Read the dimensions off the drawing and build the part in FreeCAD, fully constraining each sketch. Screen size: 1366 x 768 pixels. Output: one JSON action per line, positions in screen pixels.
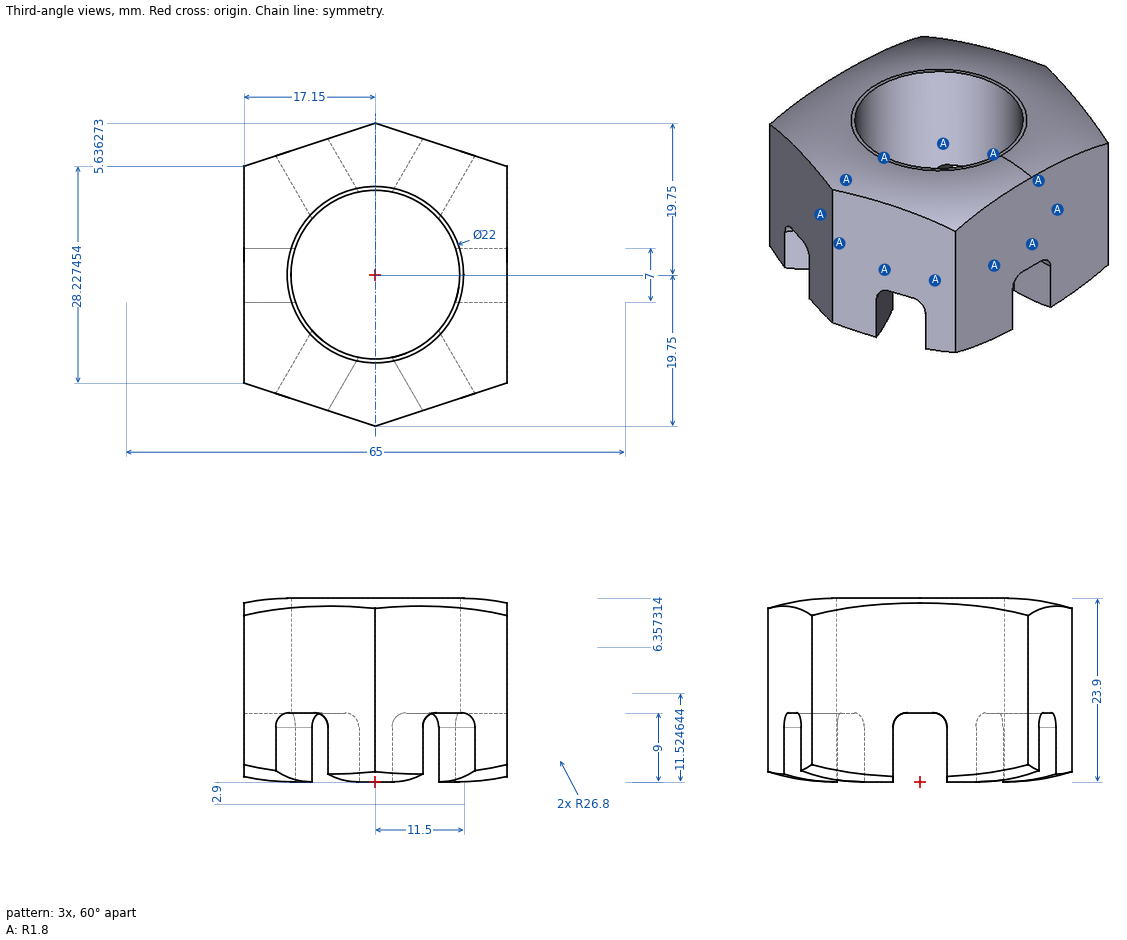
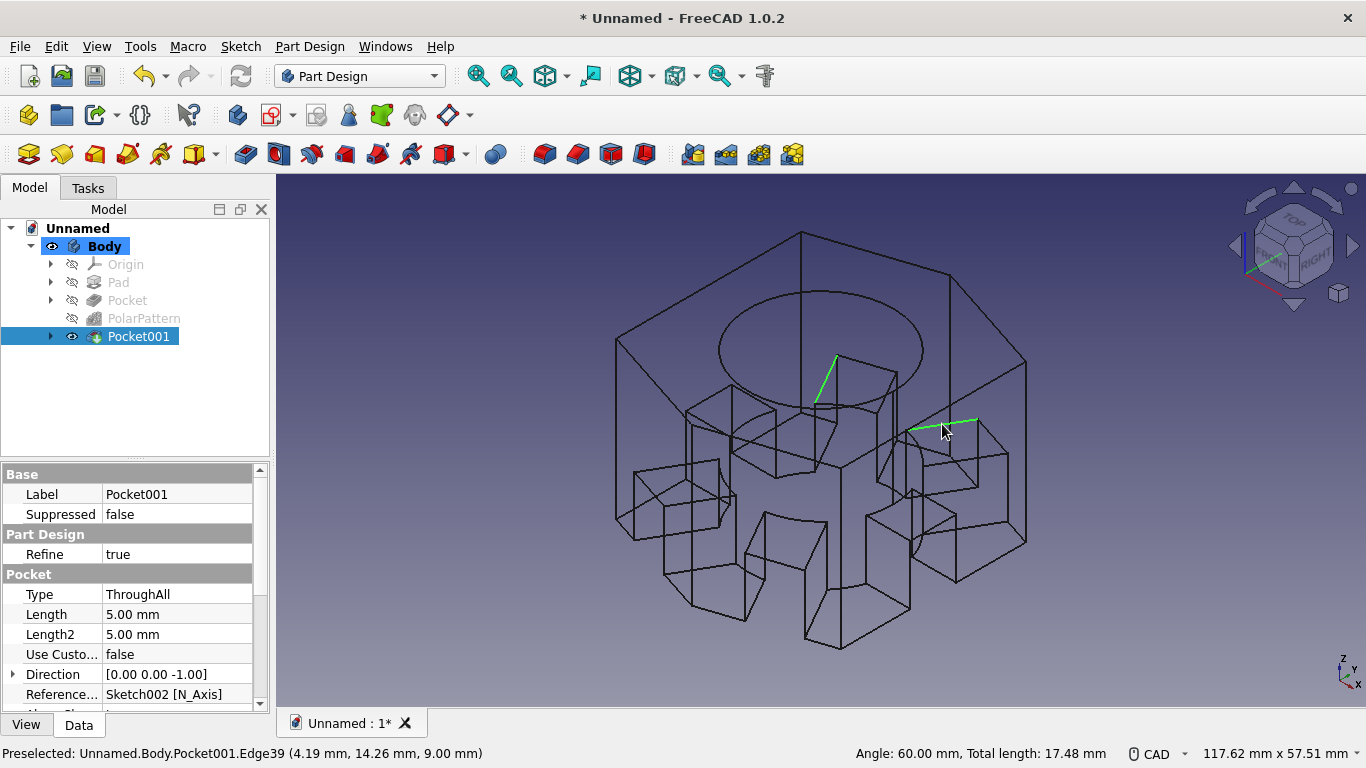
{"action": "left_click", "coordinate": [700, 500], "text": "ctrl"}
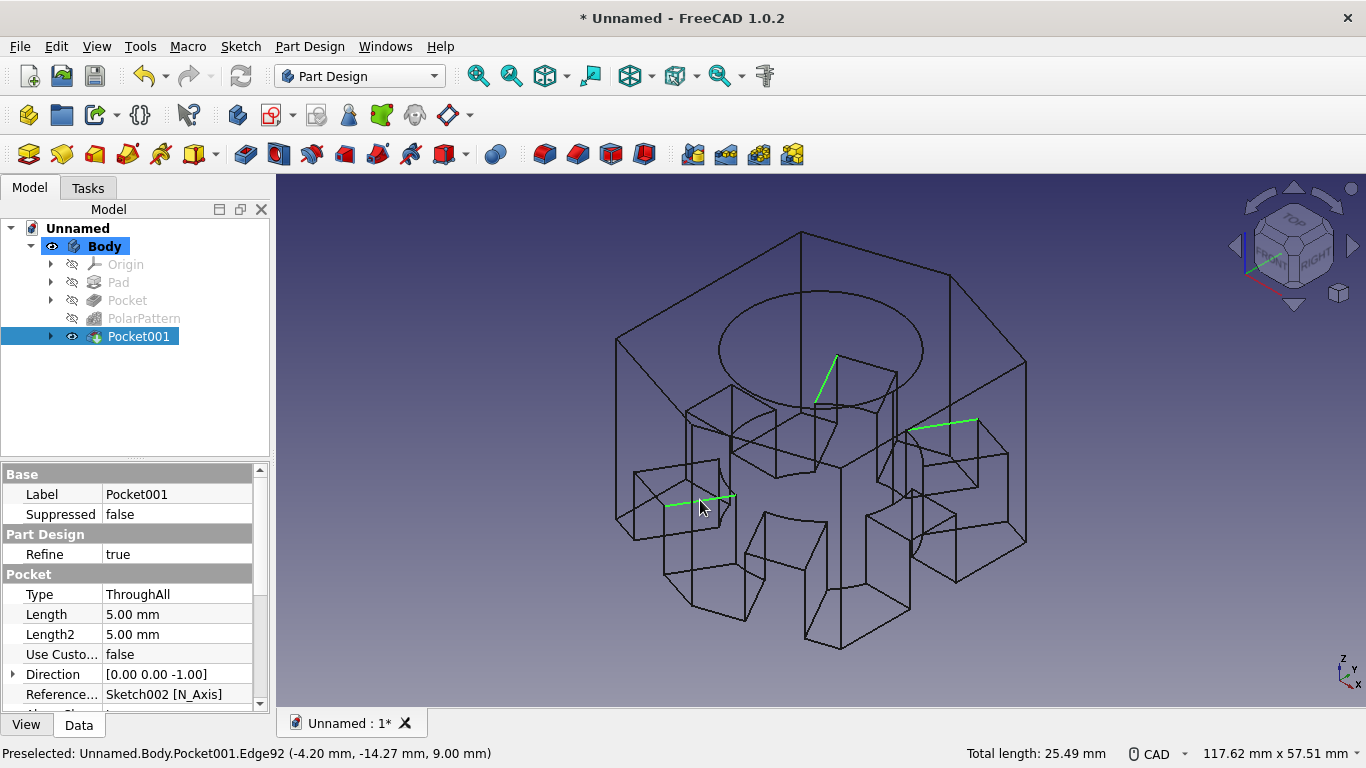
{"action": "left_click", "coordinate": [816, 545], "text": "ctrl"}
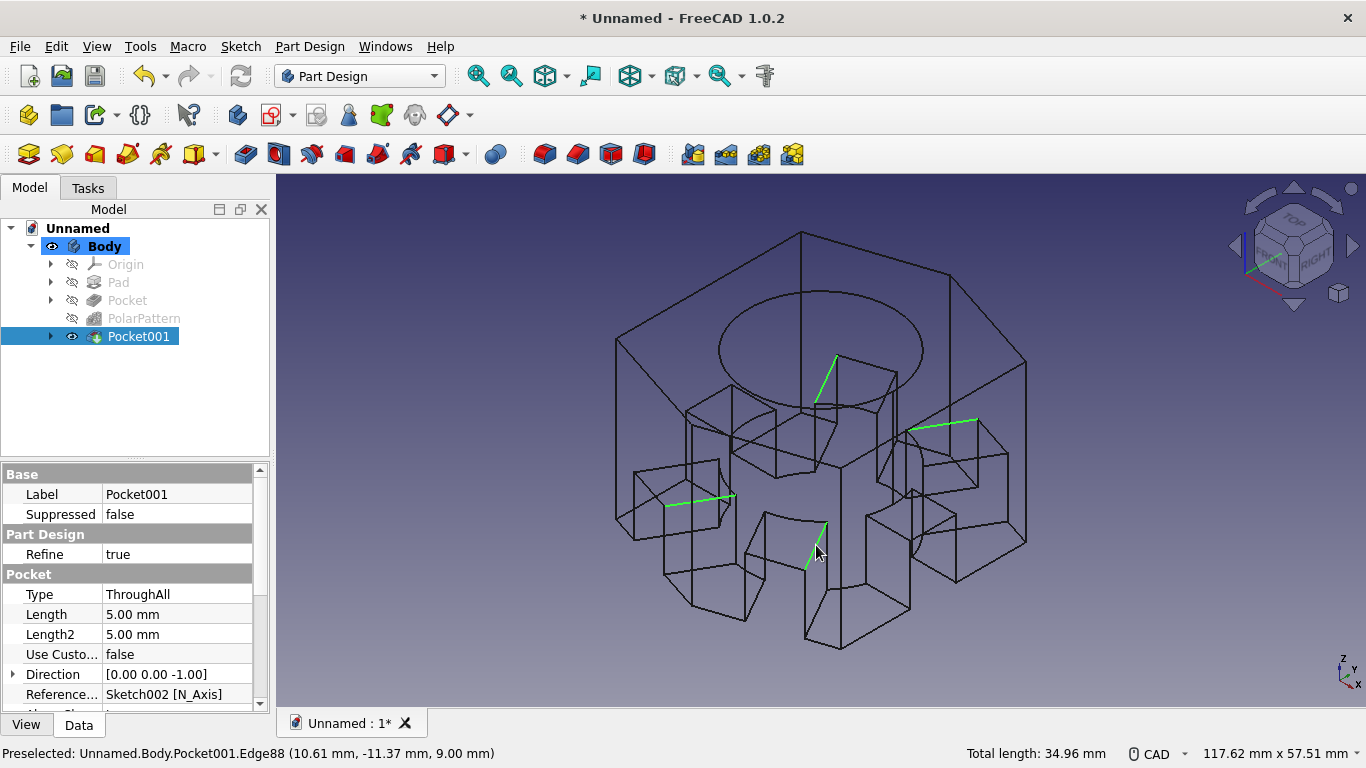
{"action": "left_click", "coordinate": [703, 420], "text": "ctrl"}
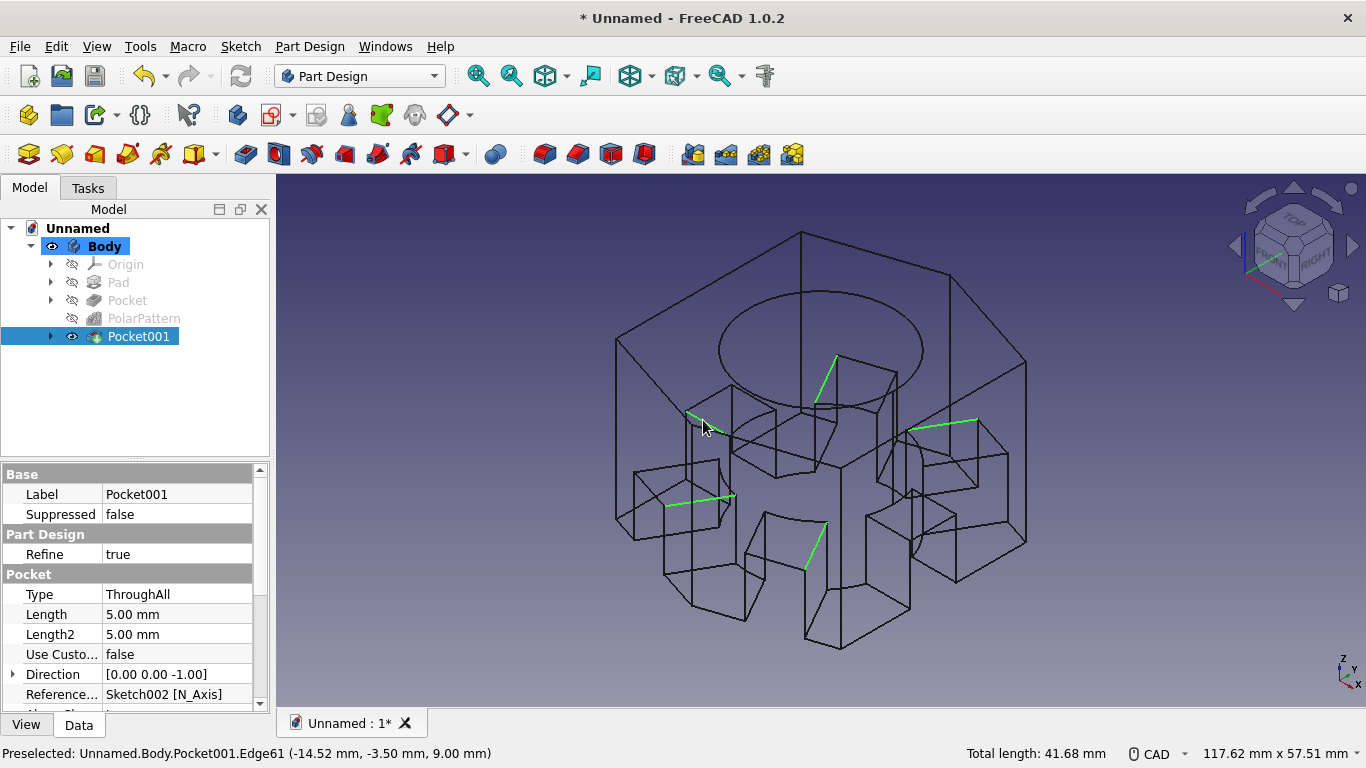
{"action": "left_click", "coordinate": [934, 501], "text": "ctrl"}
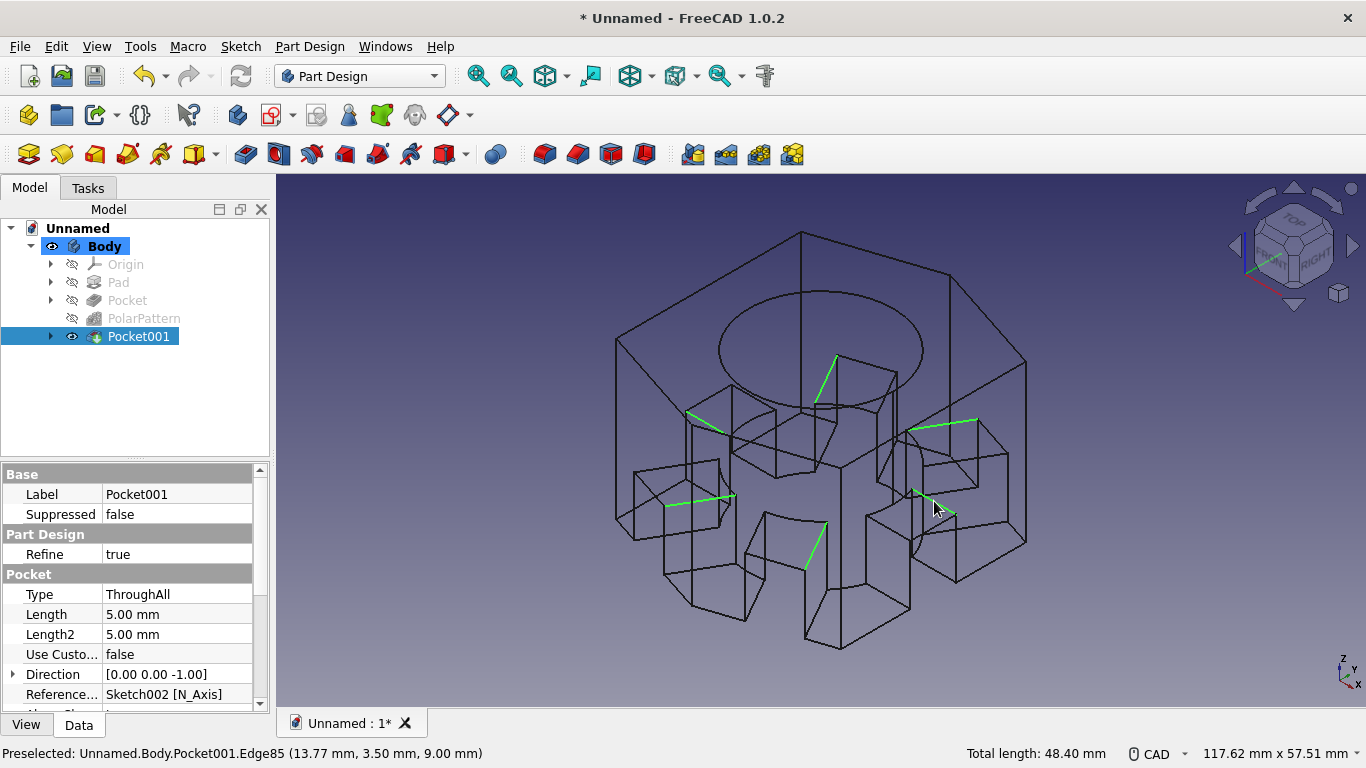
{"action": "left_click", "coordinate": [888, 527], "text": "ctrl"}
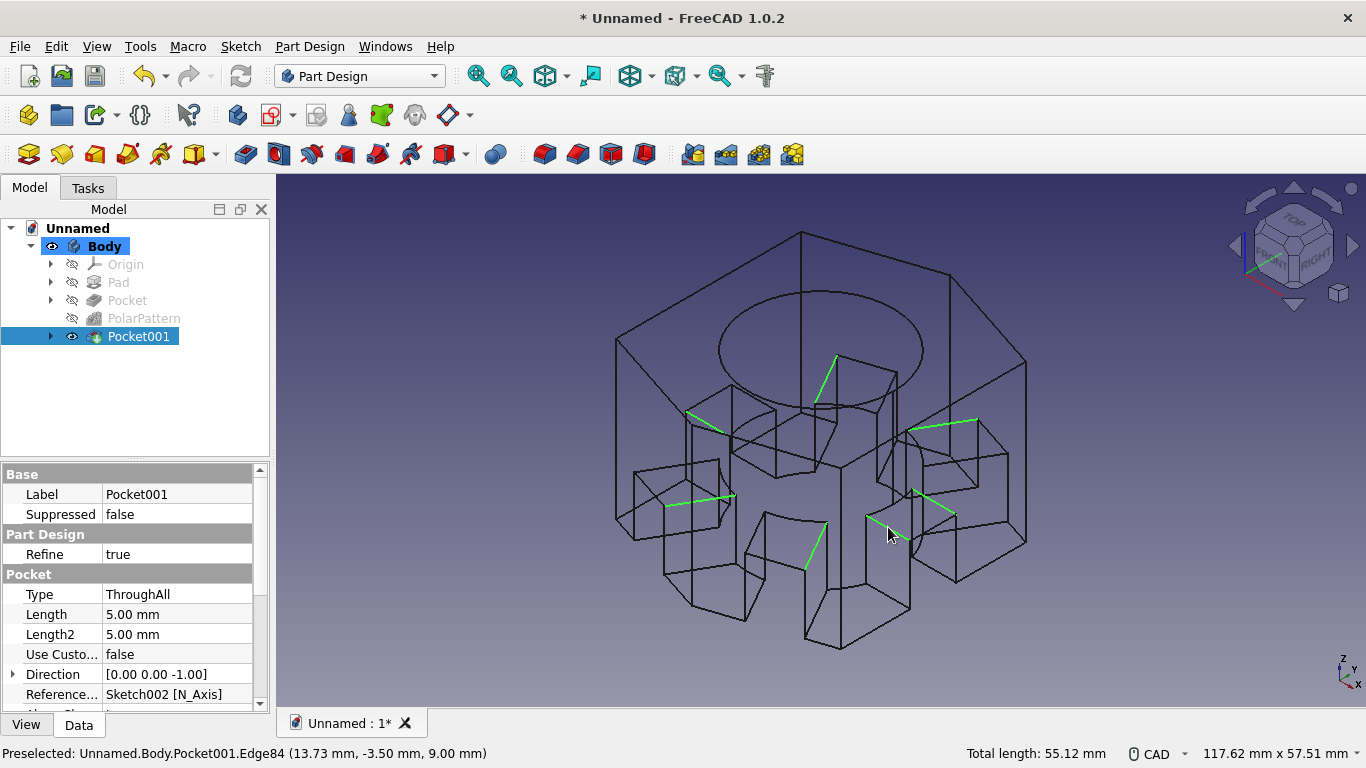
{"action": "left_click", "coordinate": [891, 384], "text": "ctrl"}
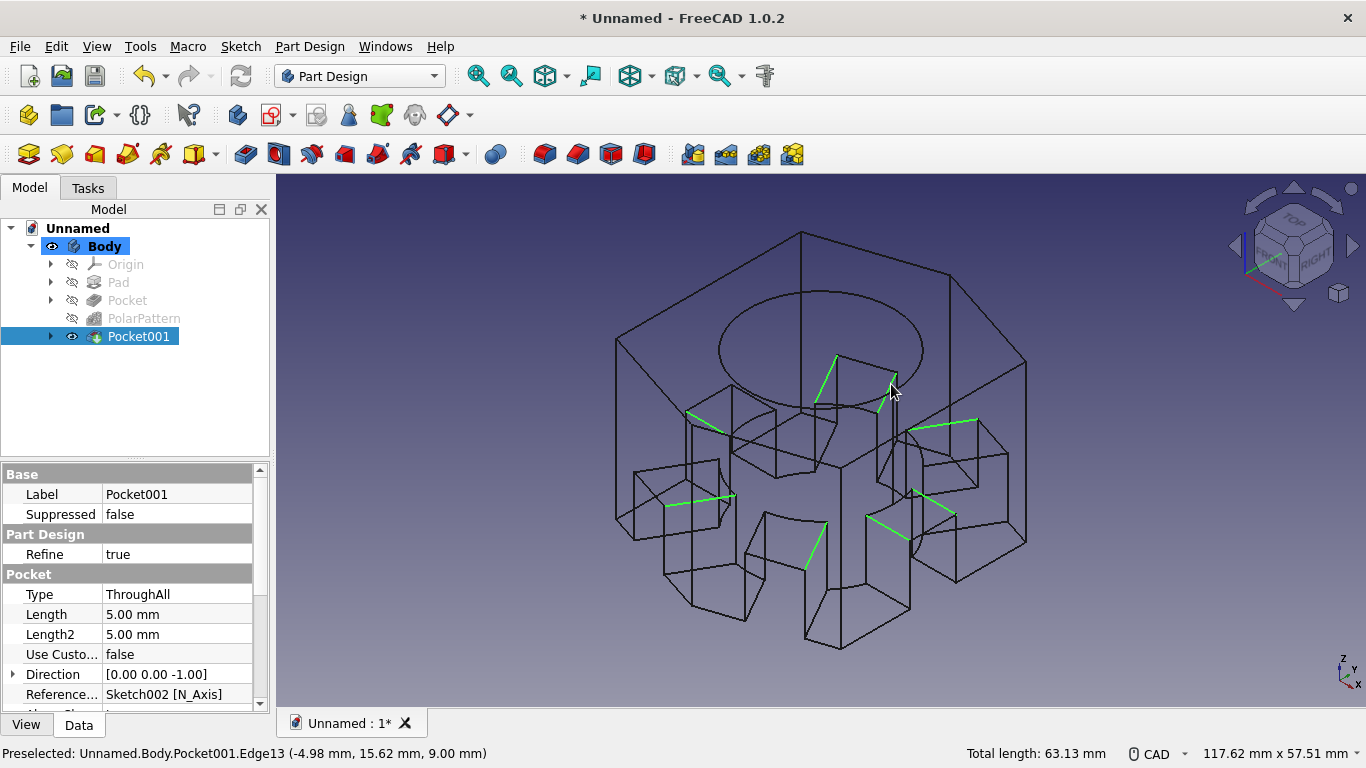
{"action": "left_click", "coordinate": [755, 532], "text": "ctrl"}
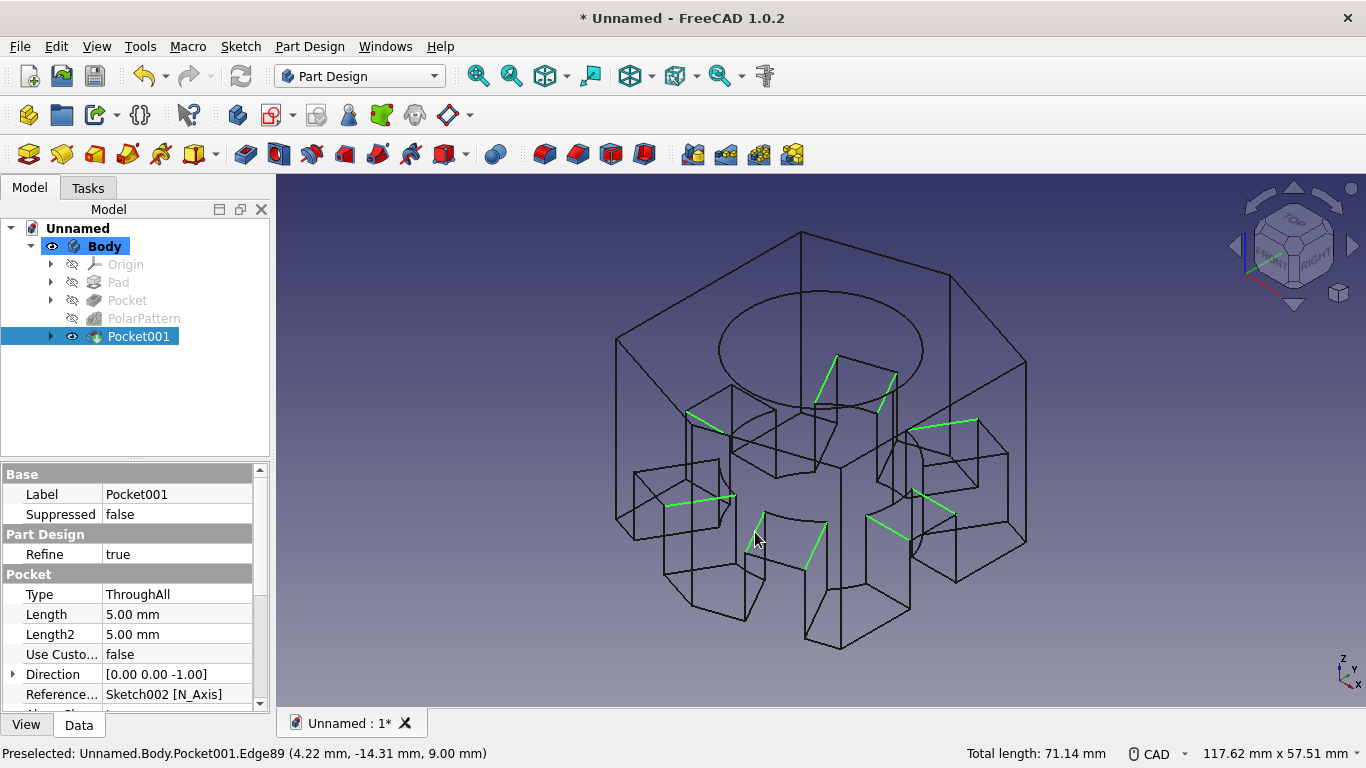
{"action": "left_click", "coordinate": [965, 459], "text": "ctrl"}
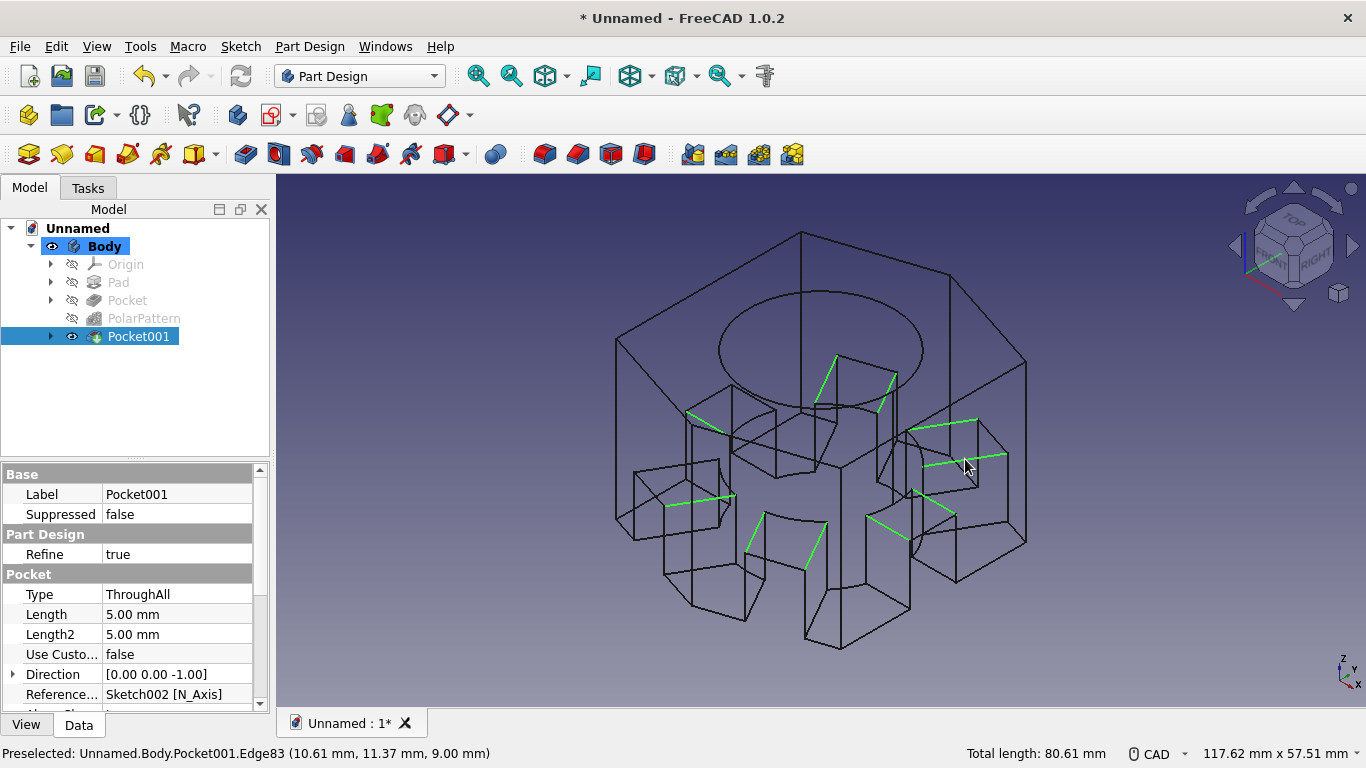
{"action": "left_click", "coordinate": [677, 465], "text": "ctrl"}